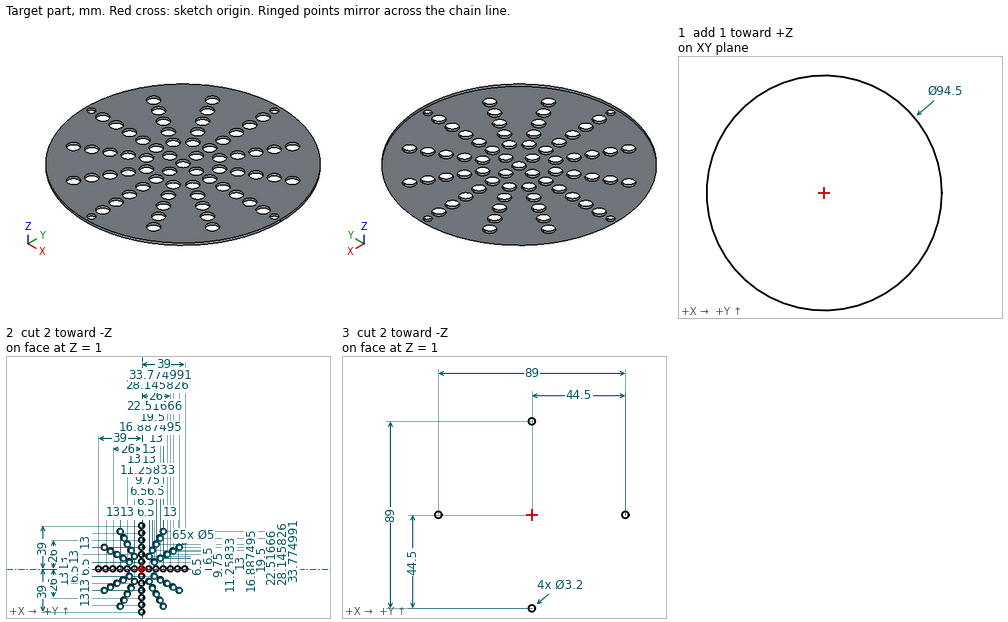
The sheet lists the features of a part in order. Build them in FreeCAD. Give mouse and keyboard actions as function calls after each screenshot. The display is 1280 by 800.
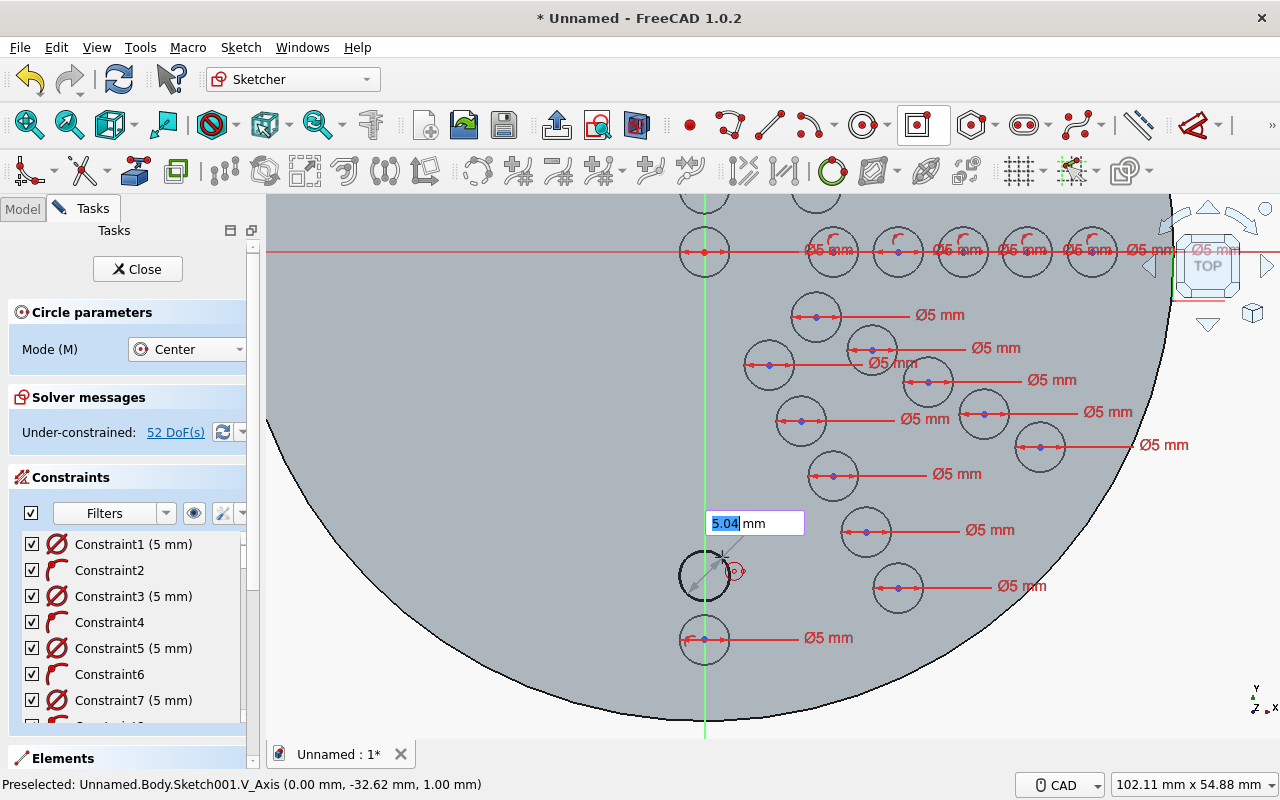
text(5)
key(Return)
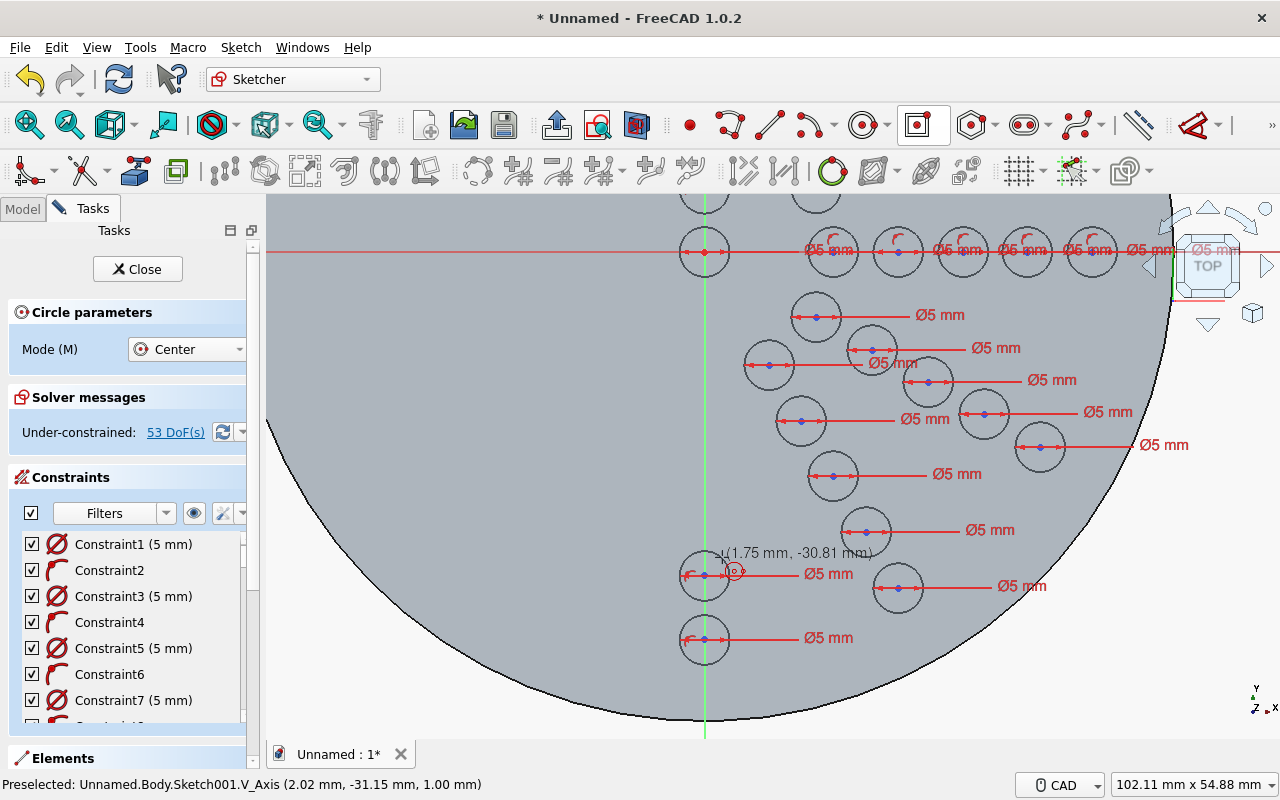
click(705, 510)
move(722, 493)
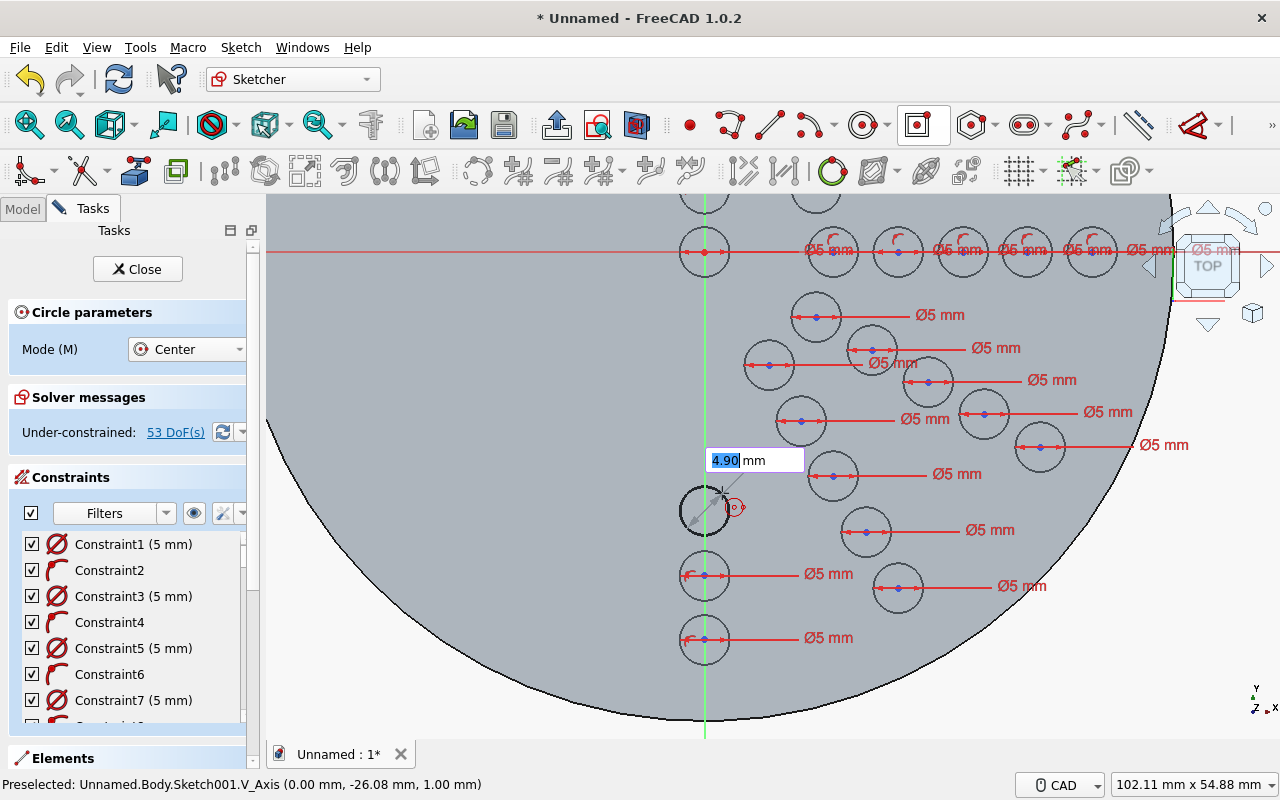
text(5)
key(Return)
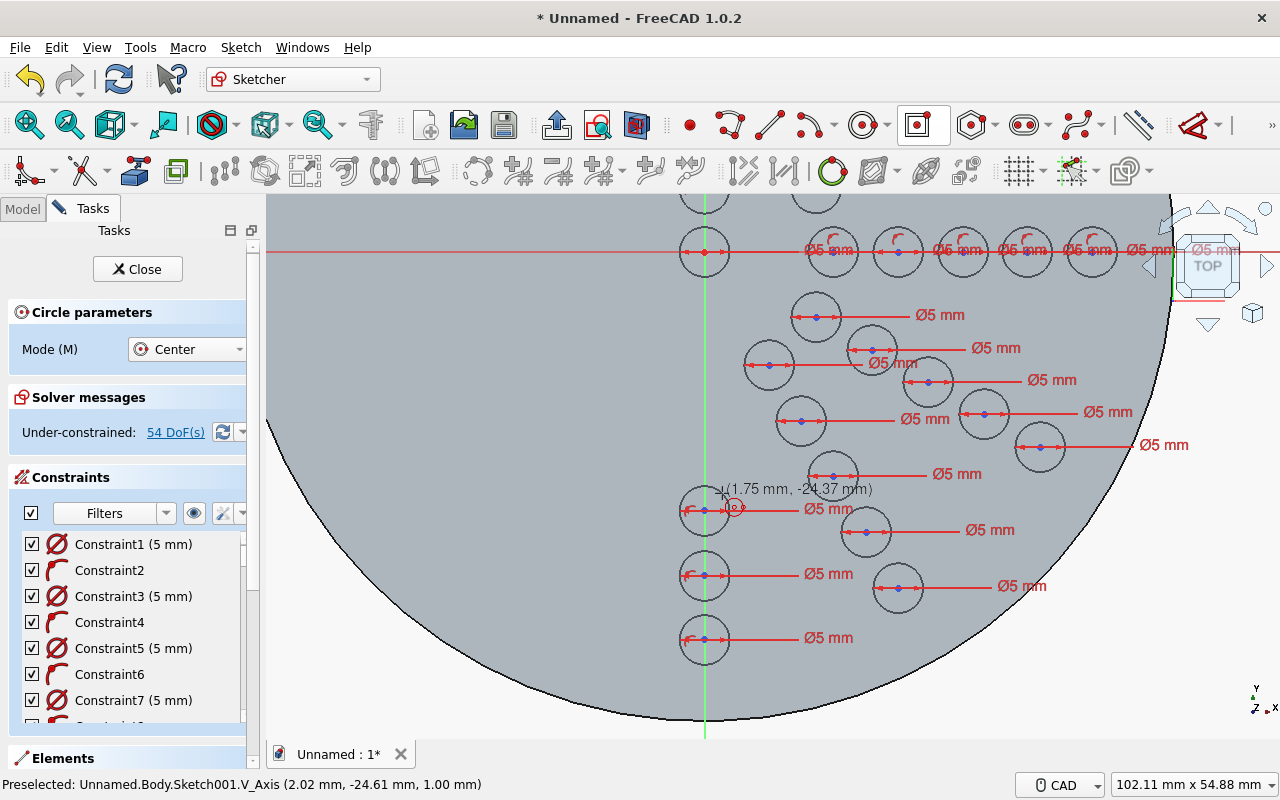
click(705, 446)
move(722, 428)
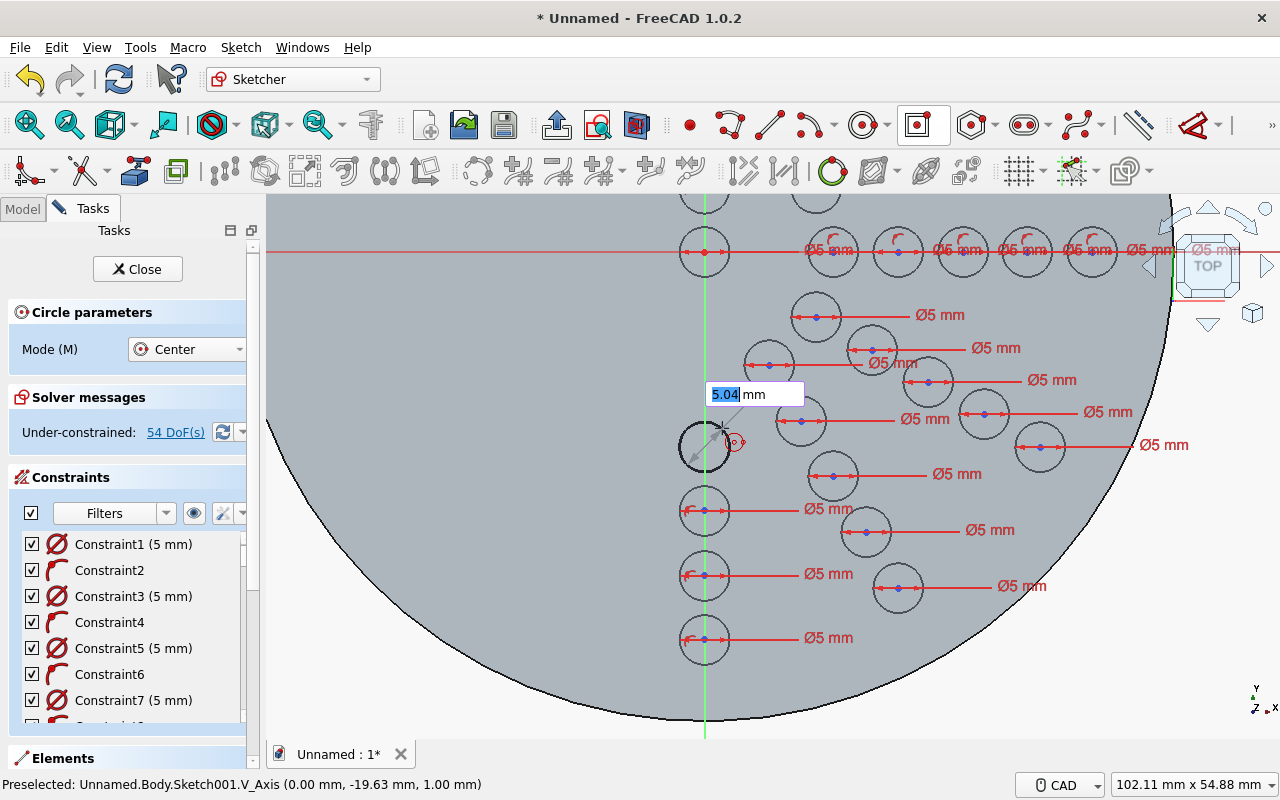
text(5)
key(Return)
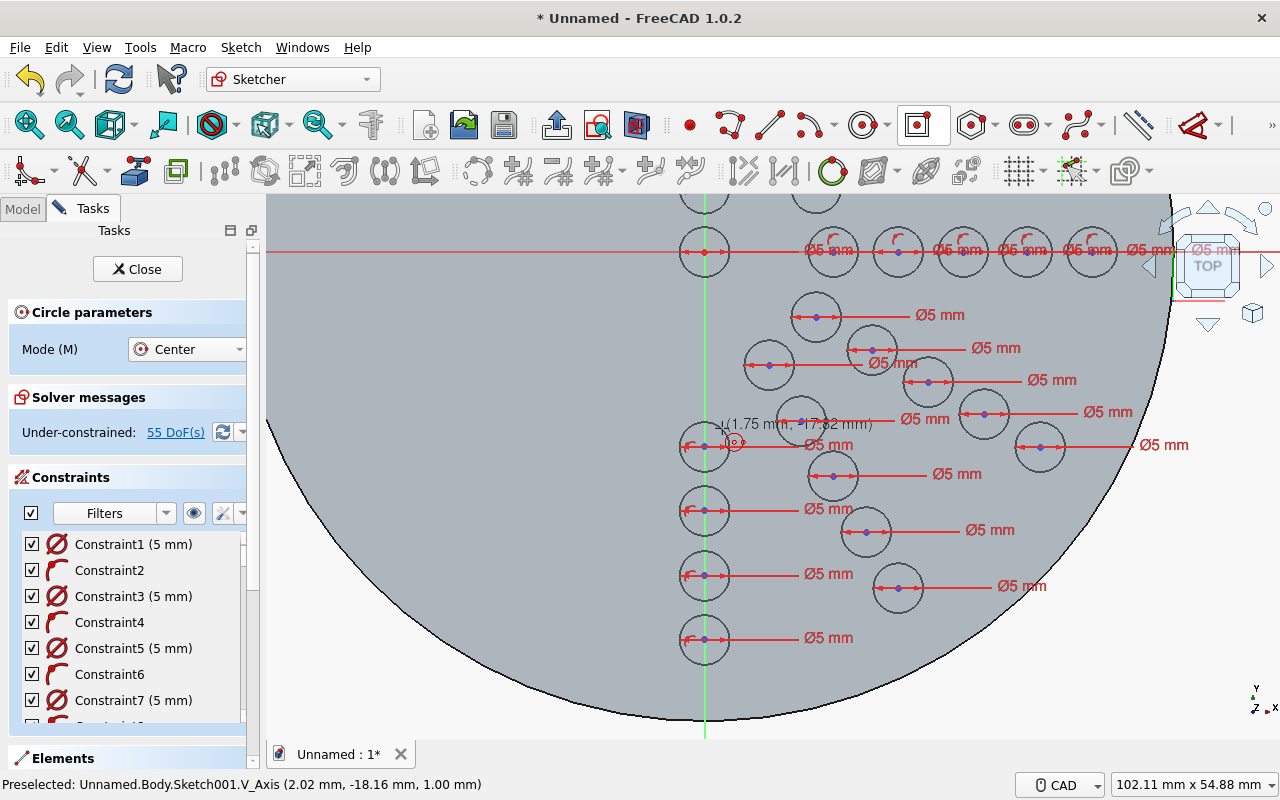
click(705, 381)
move(722, 364)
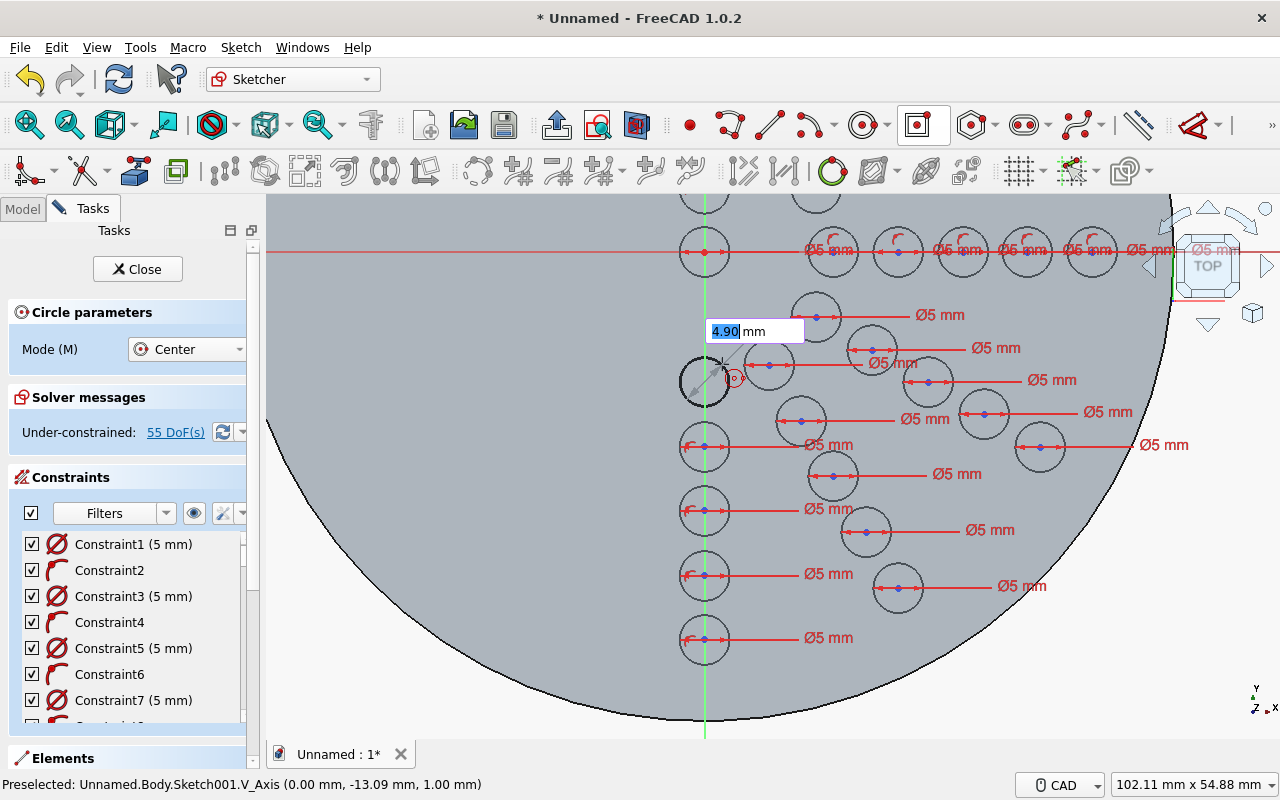
text(5)
key(Return)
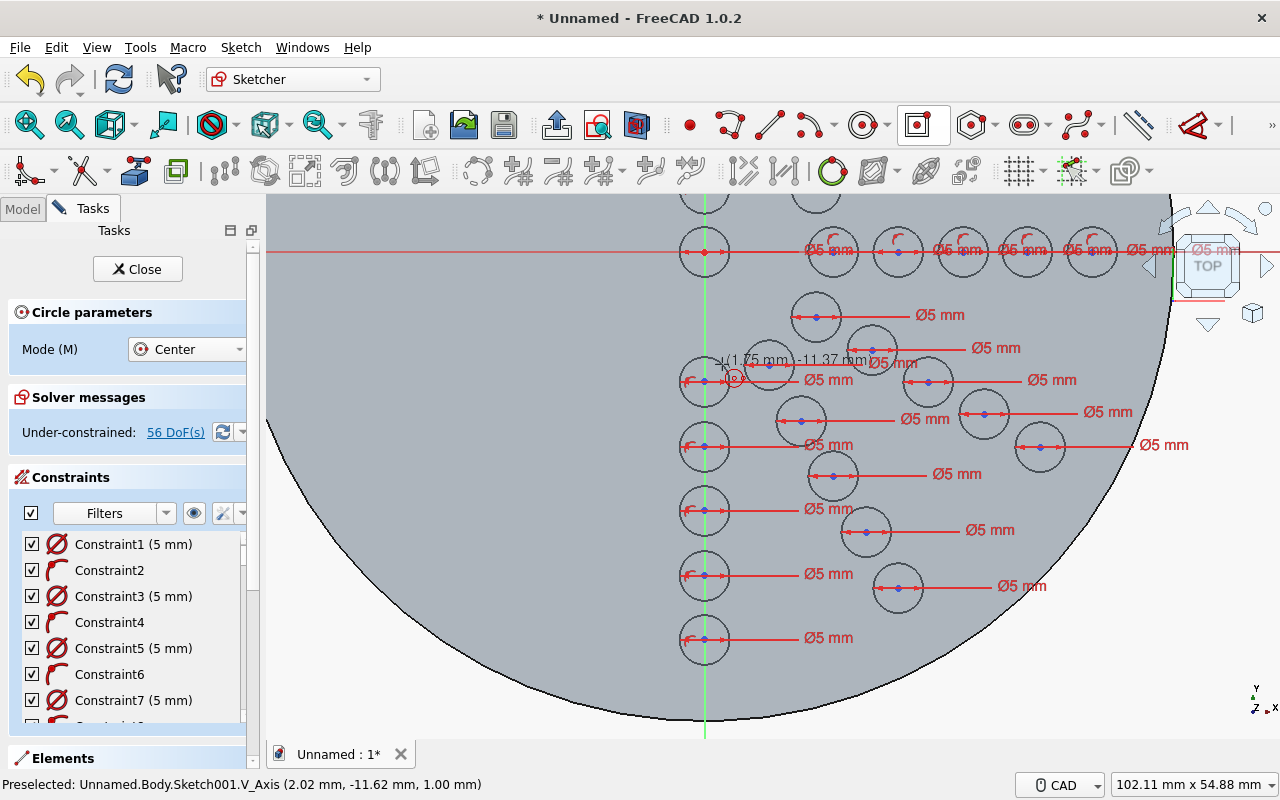
click(511, 587)
move(528, 570)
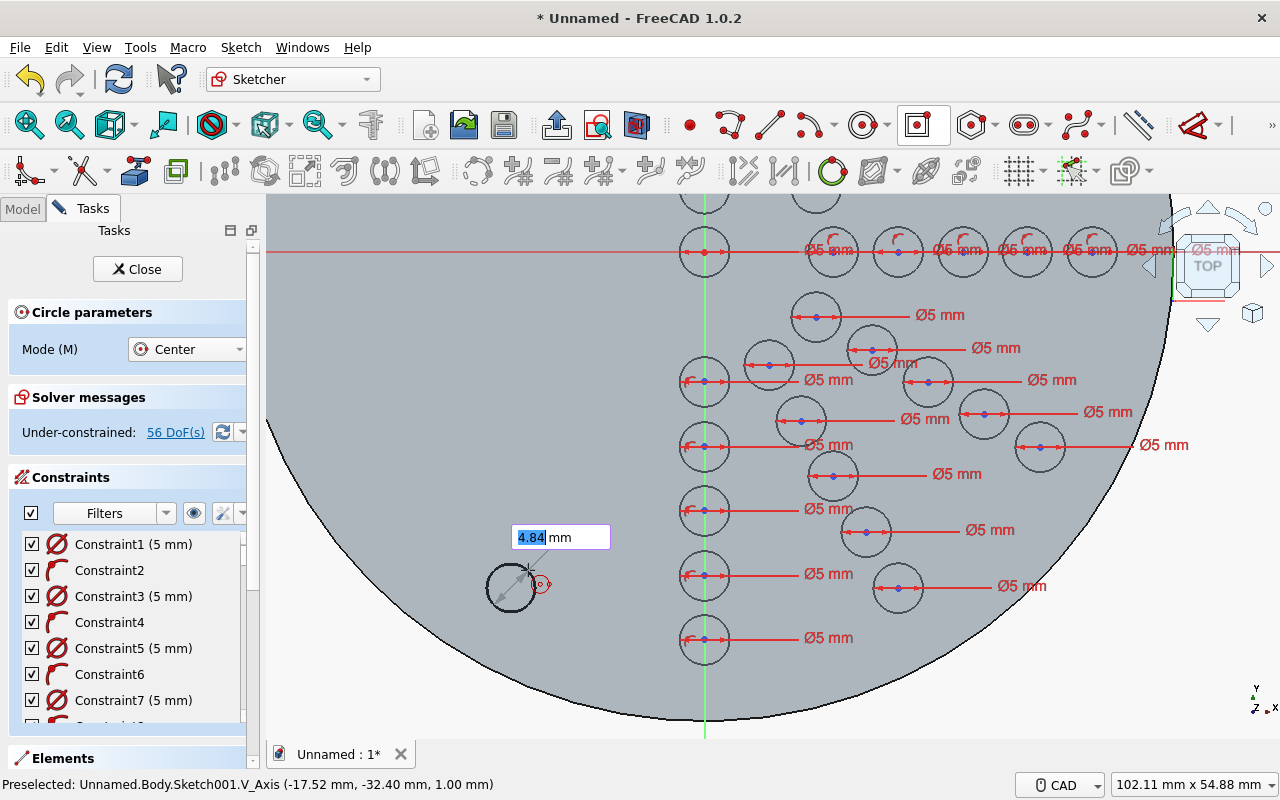
text(5)
key(Return)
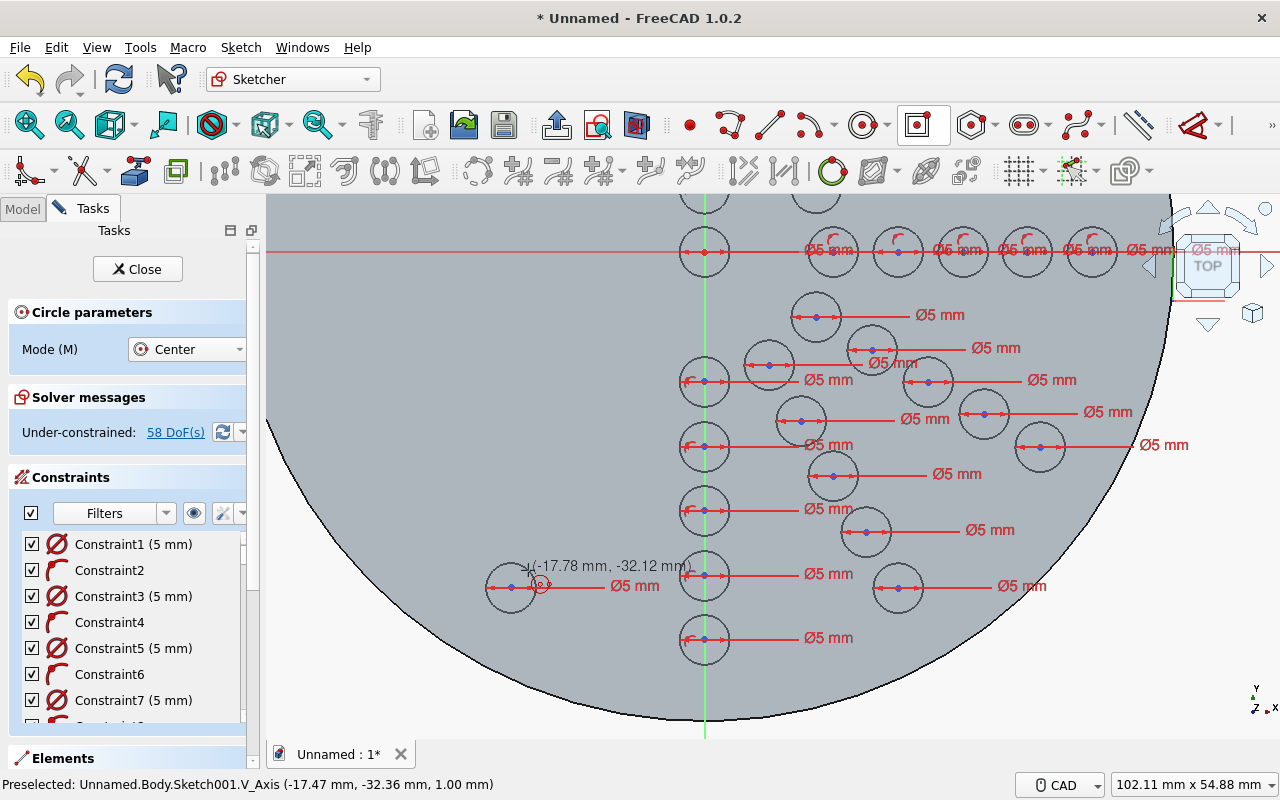
click(543, 532)
move(561, 514)